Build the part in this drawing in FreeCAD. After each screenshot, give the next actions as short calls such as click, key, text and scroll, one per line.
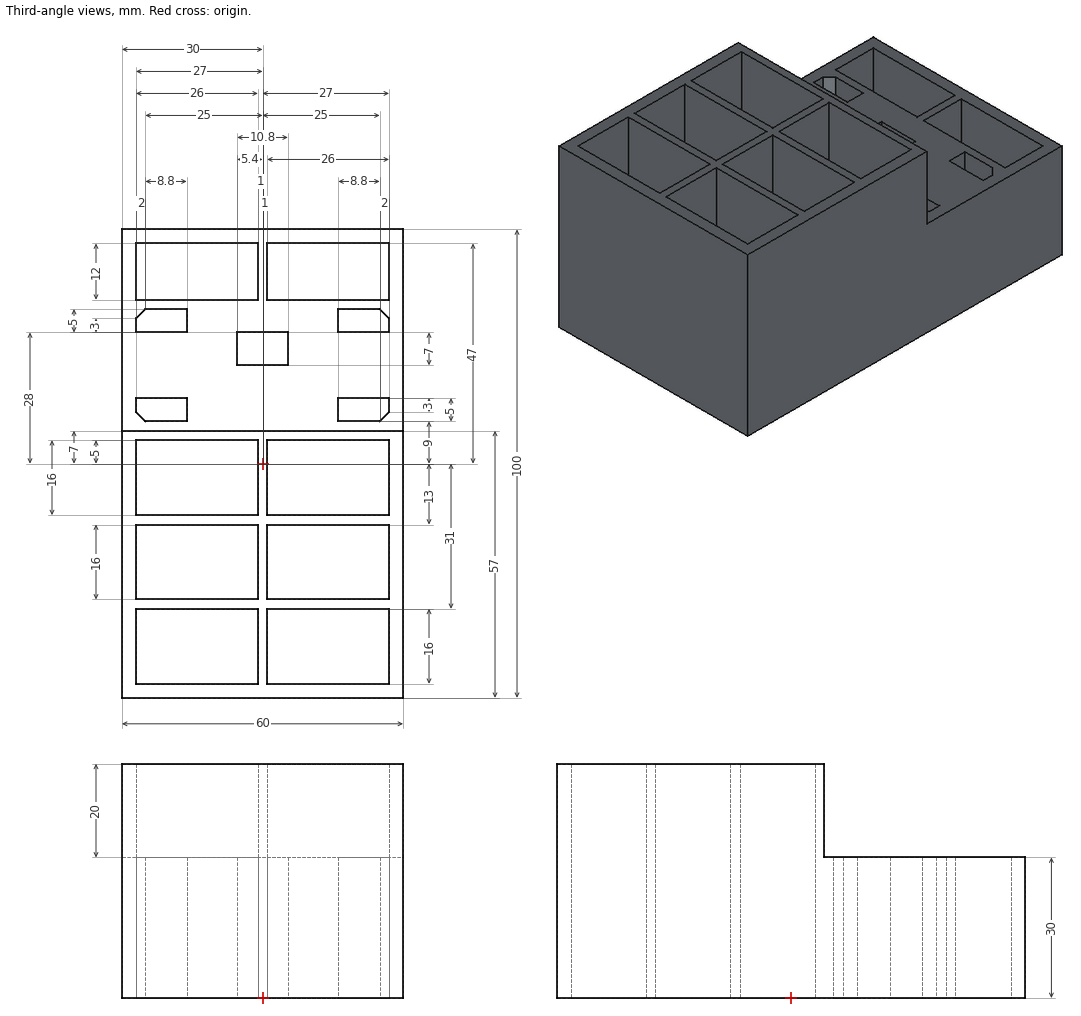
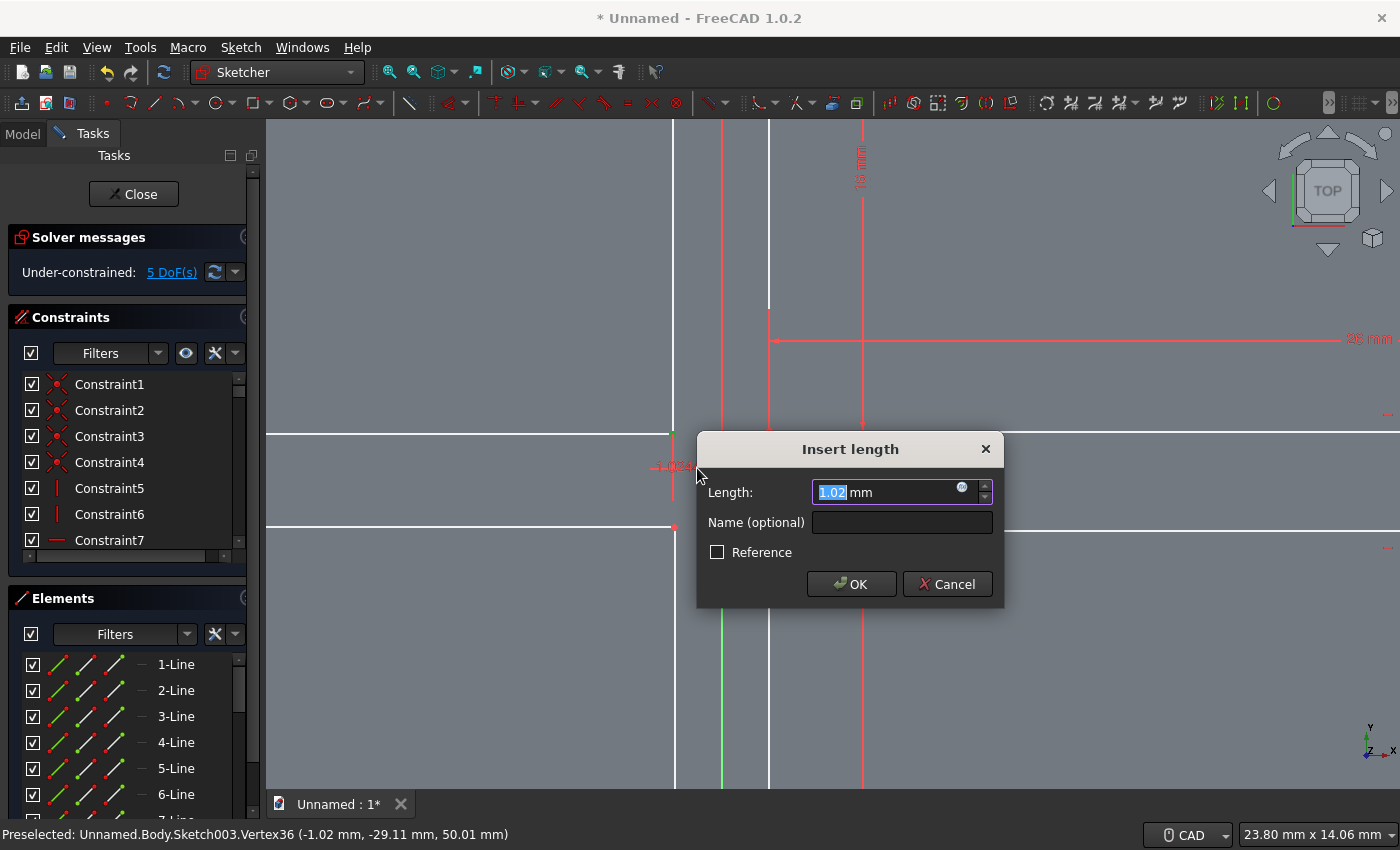
text(1)
key(Return)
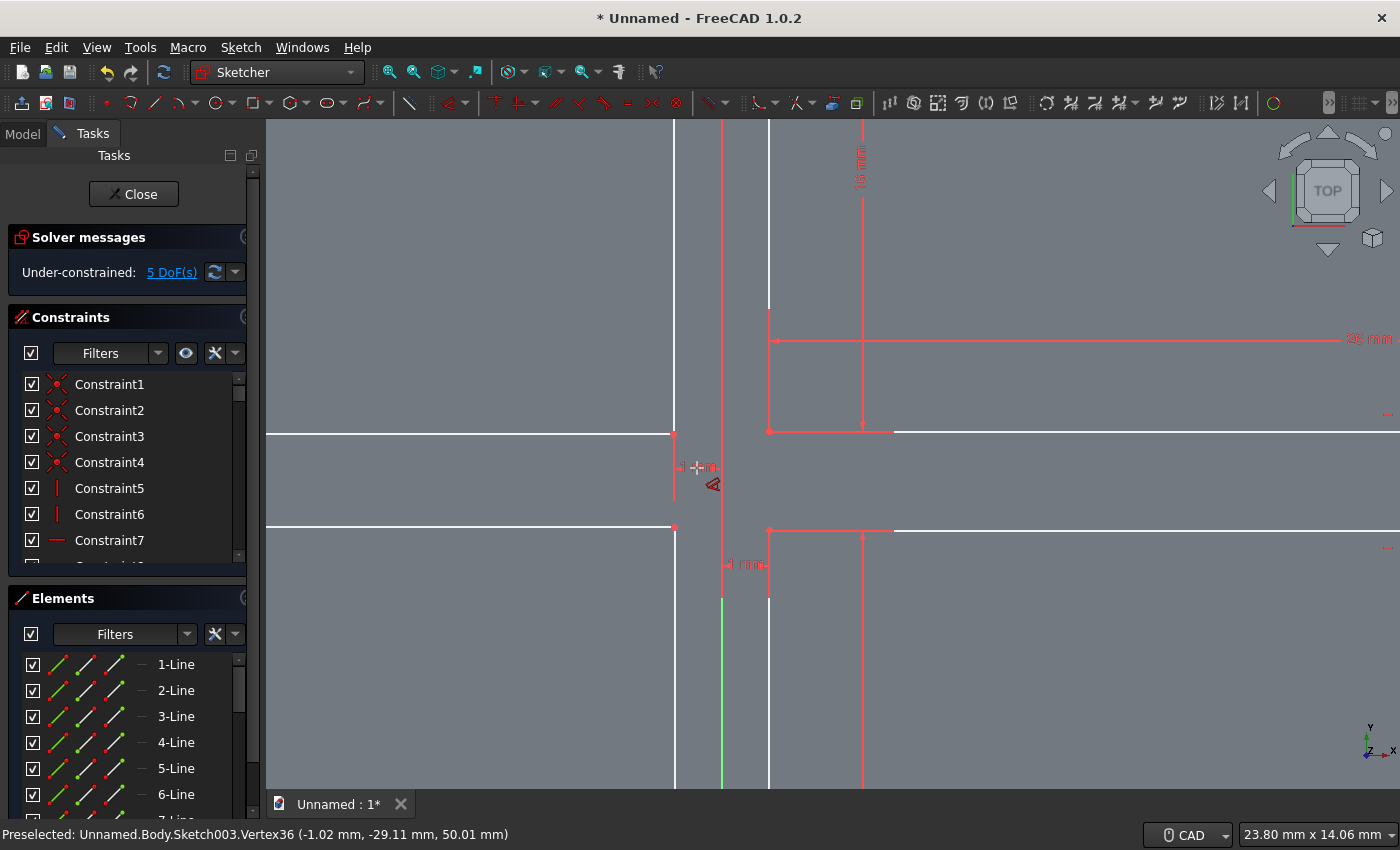
scroll(773, 534, down, 9)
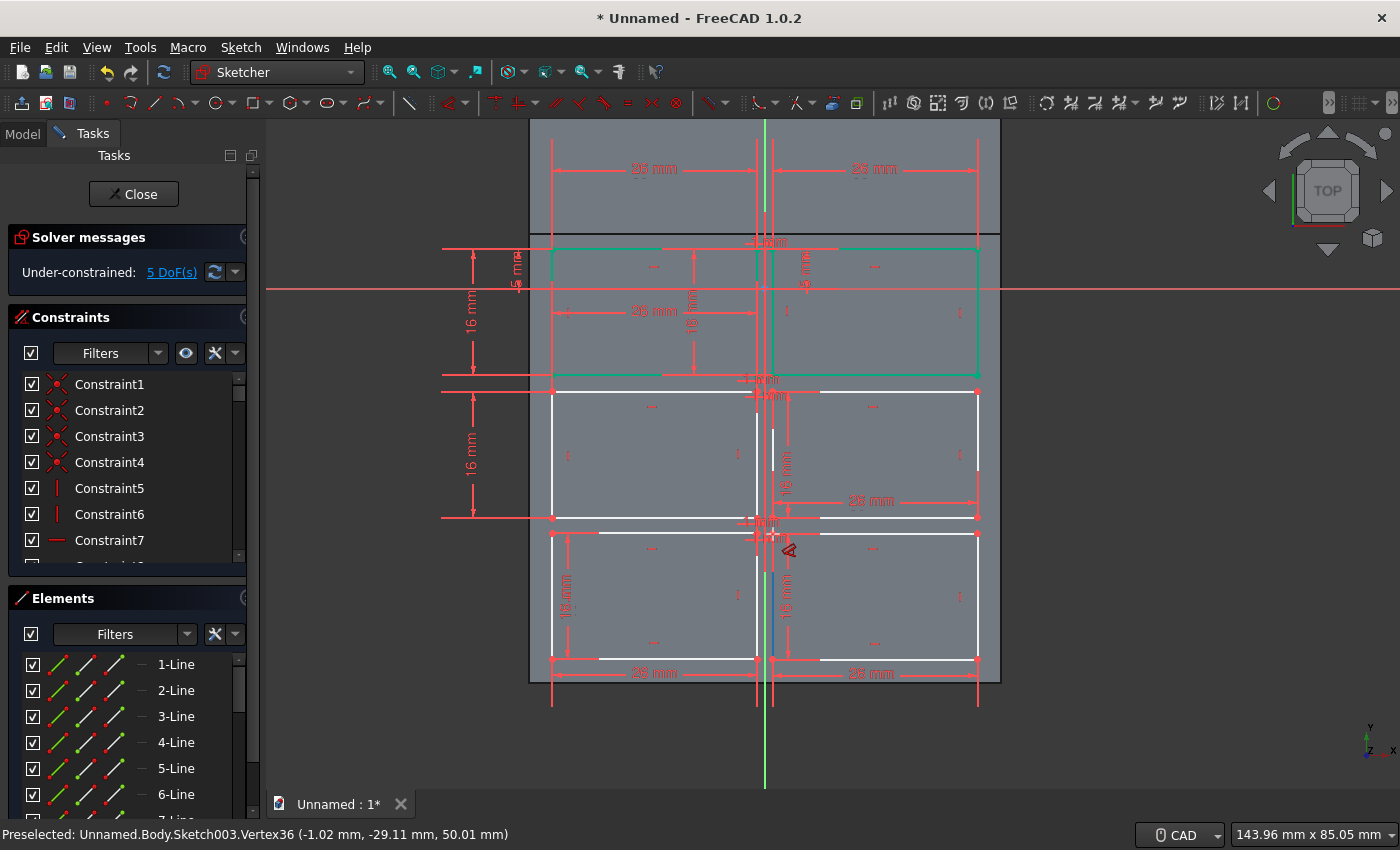
scroll(757, 659, up, 9)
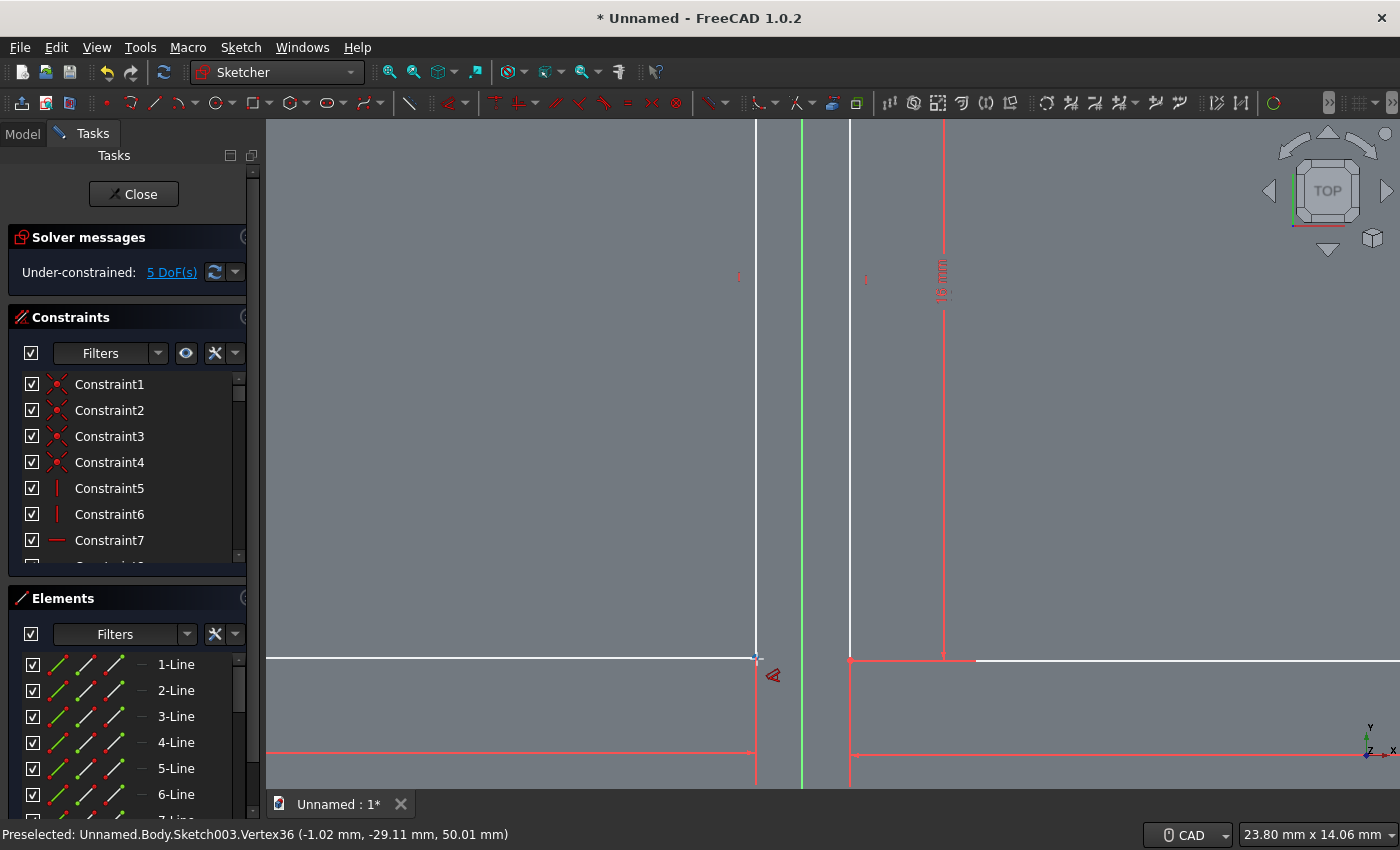
click(756, 658)
click(779, 692)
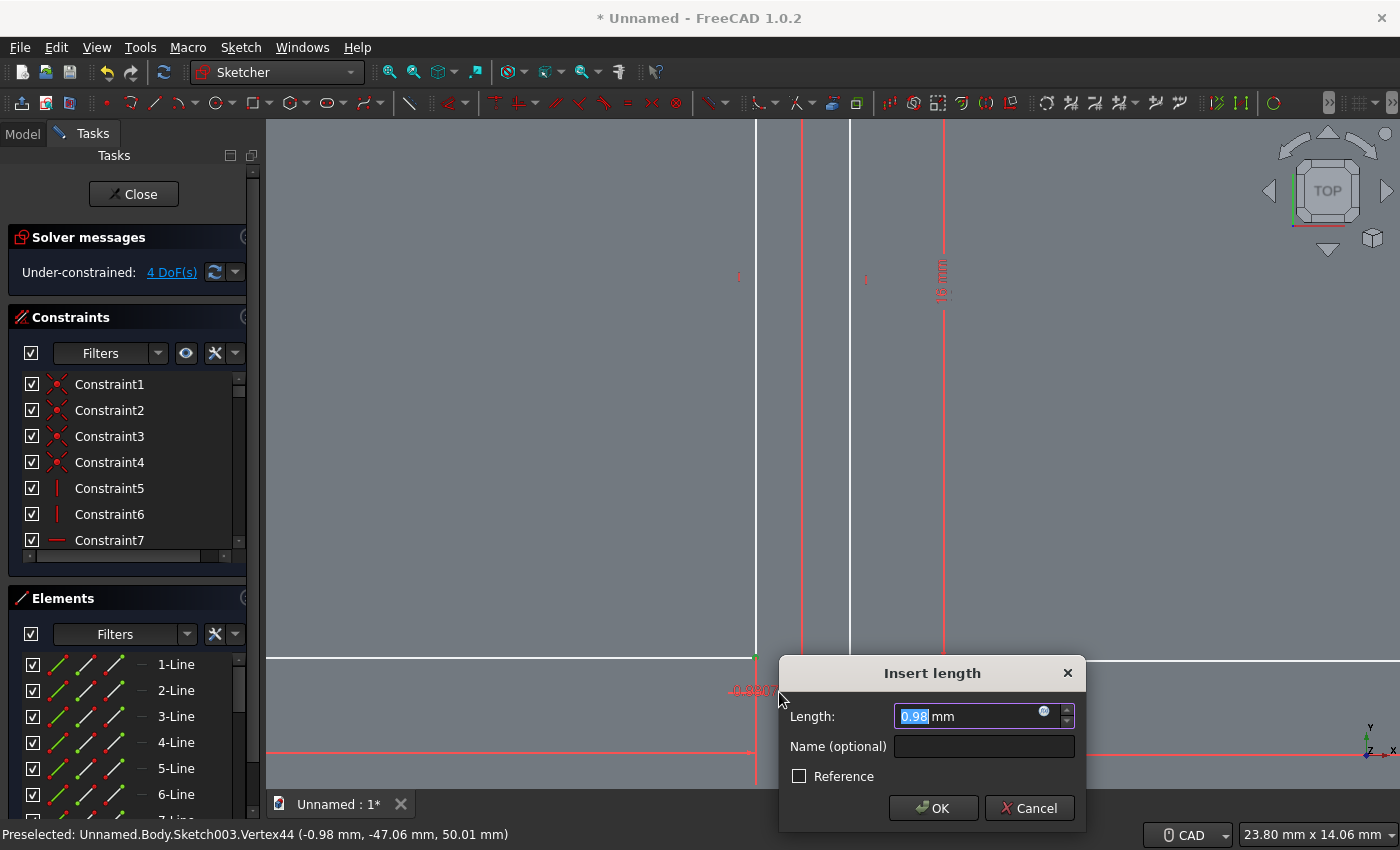
text(1)
key(Return)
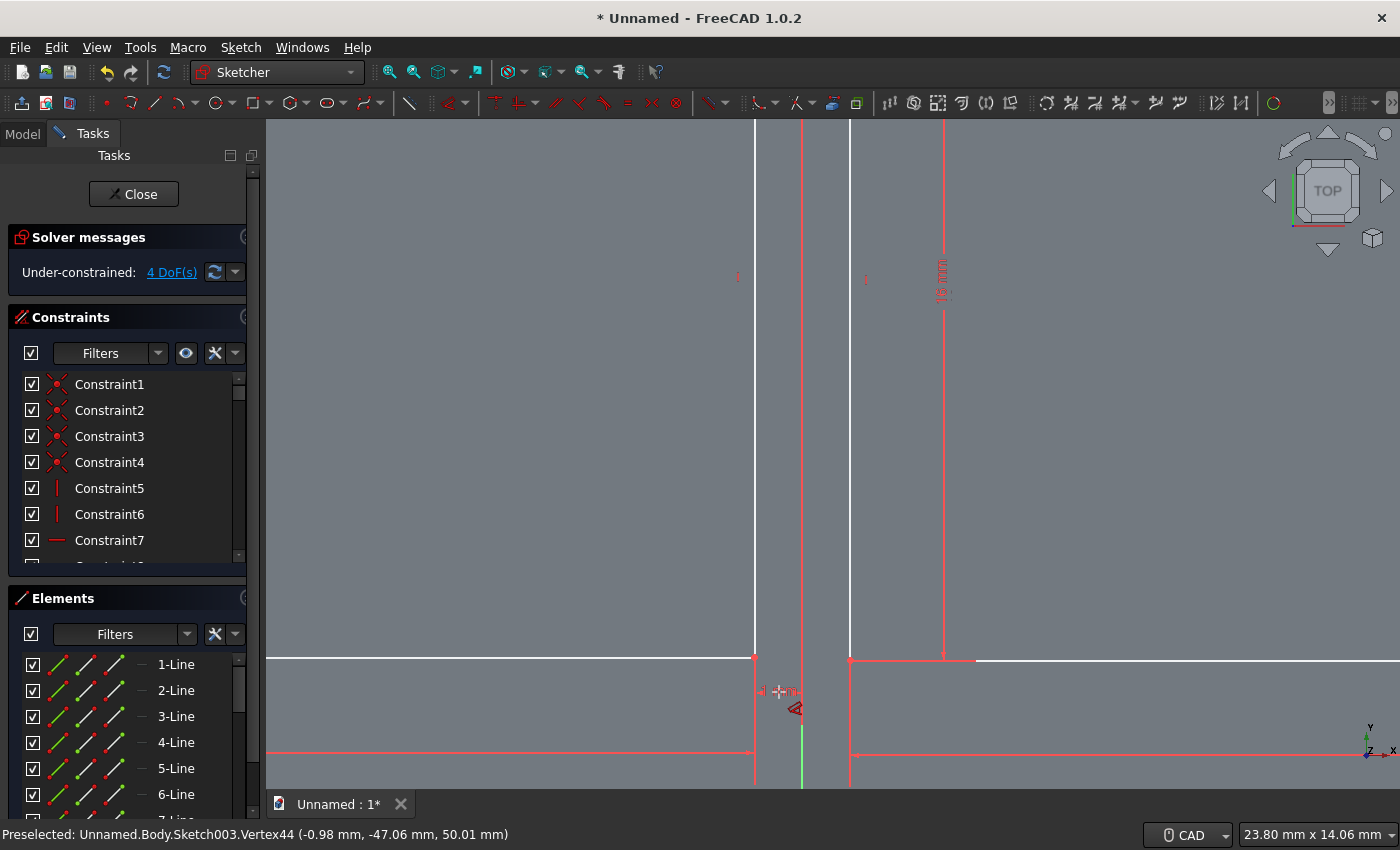
scroll(757, 660, down, 9)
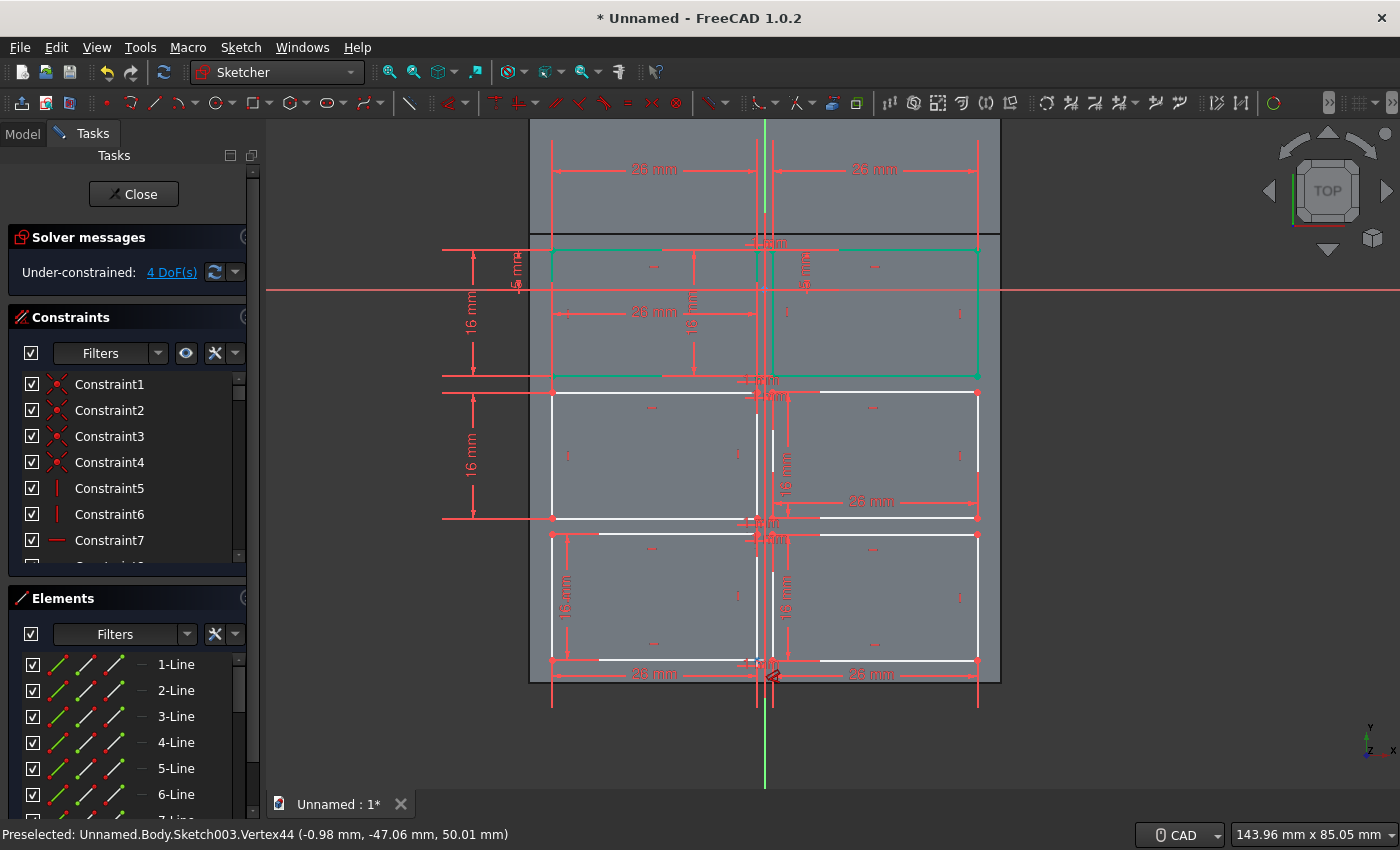
click(773, 392)
click(807, 341)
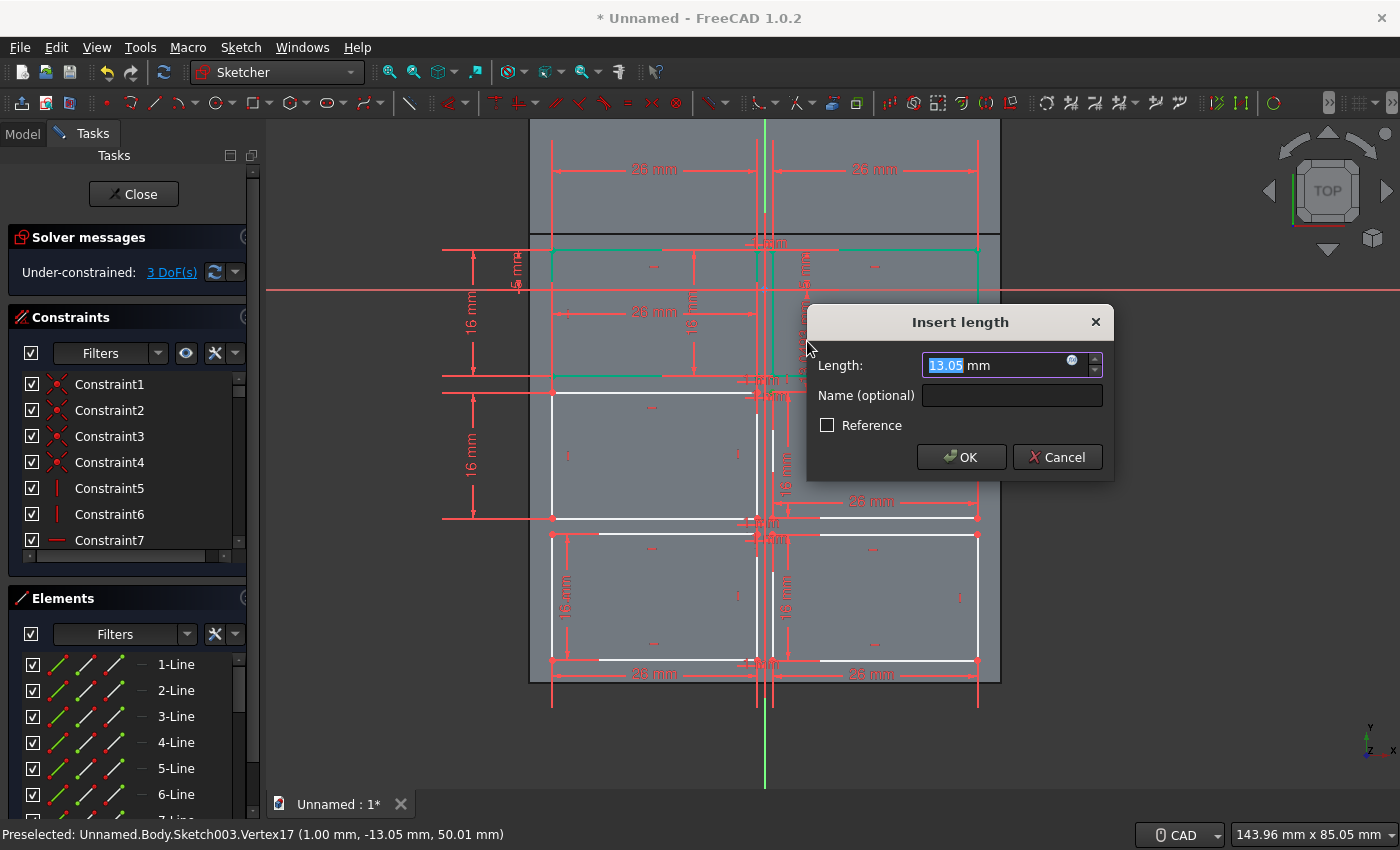
text(13)
key(Return)